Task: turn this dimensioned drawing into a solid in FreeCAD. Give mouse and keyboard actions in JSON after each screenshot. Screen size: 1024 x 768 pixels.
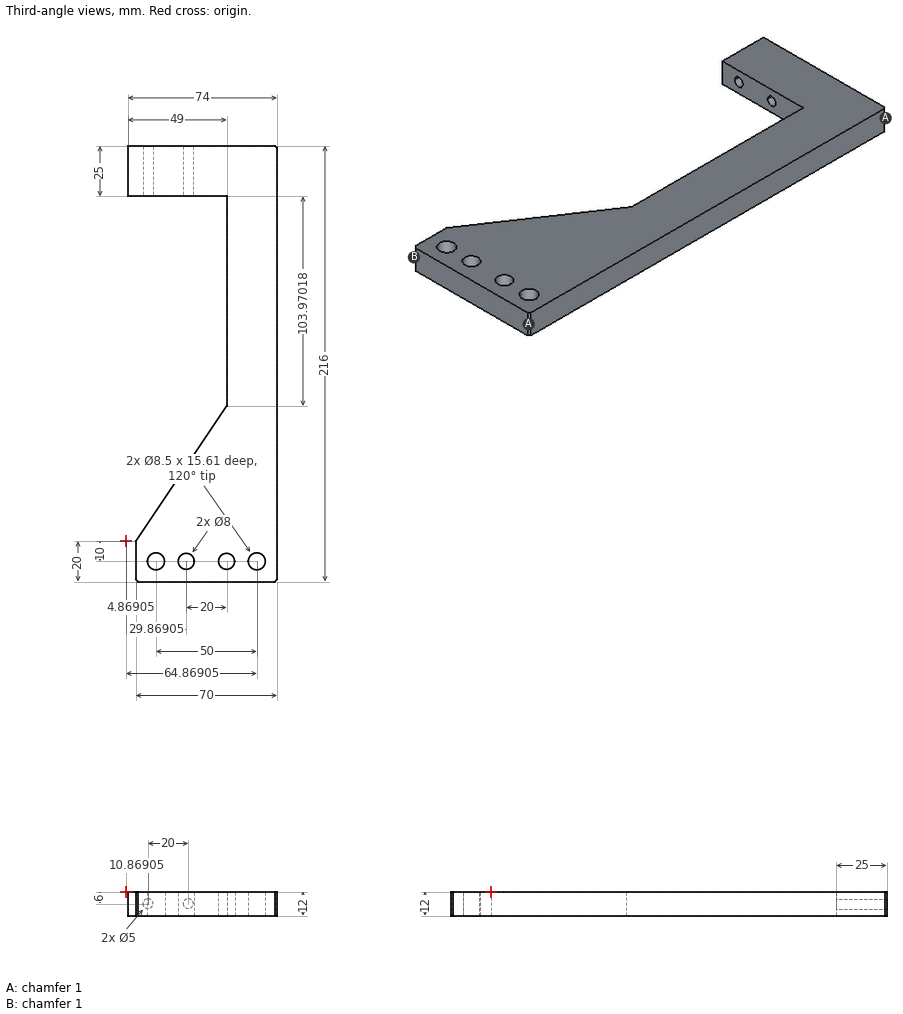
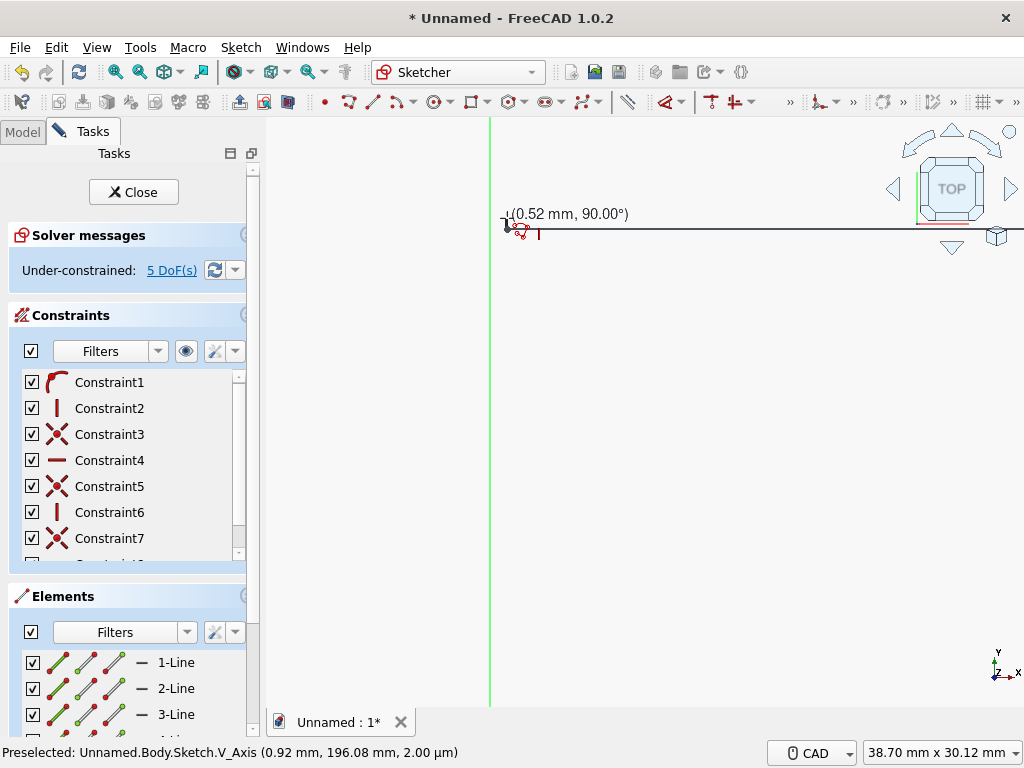
{"action": "scroll", "coordinate": [512, 220], "scroll_direction": "down", "scroll_amount": 12}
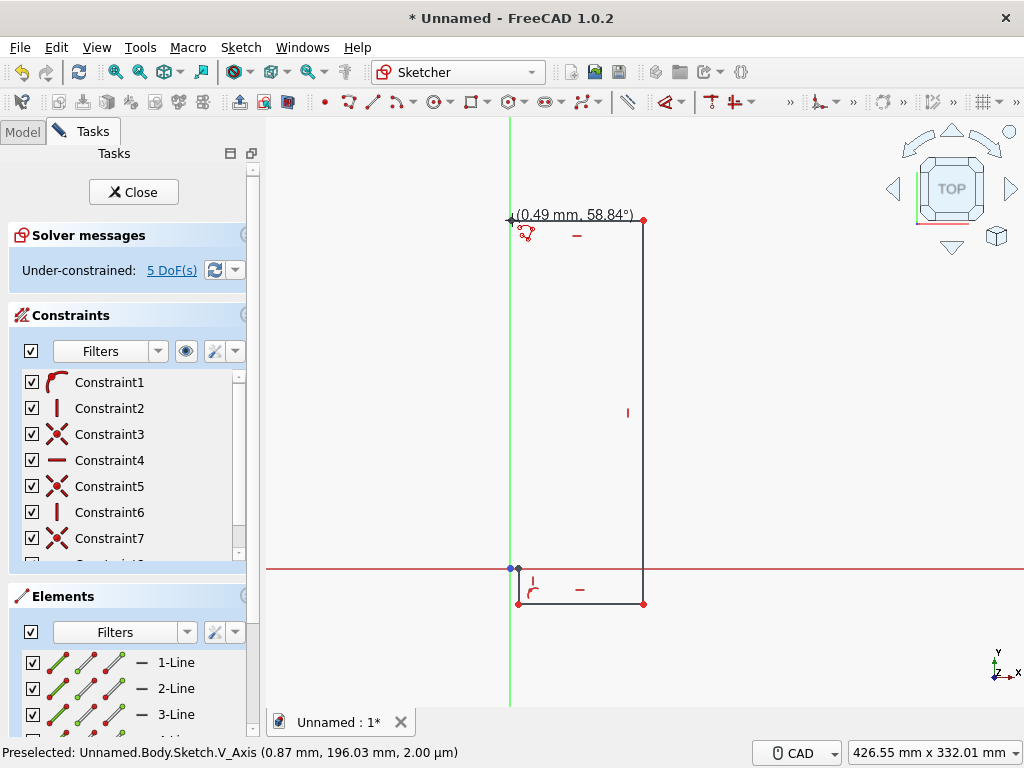
{"action": "scroll", "coordinate": [512, 265], "scroll_direction": "up", "scroll_amount": 12}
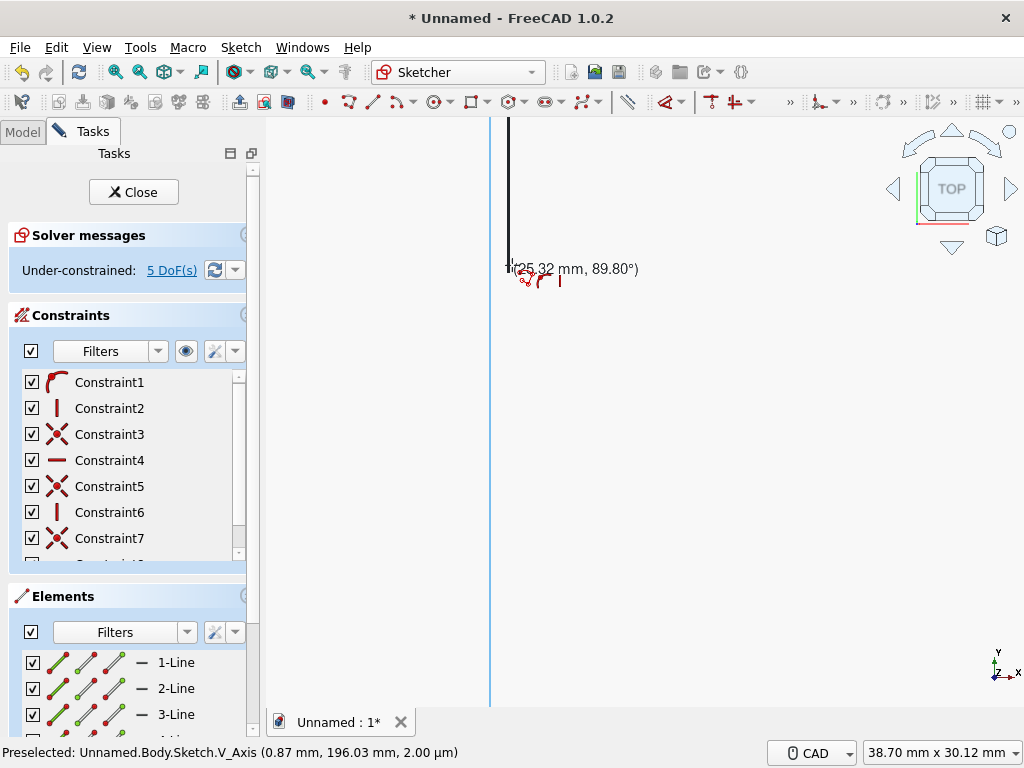
{"action": "left_click", "coordinate": [507, 259]}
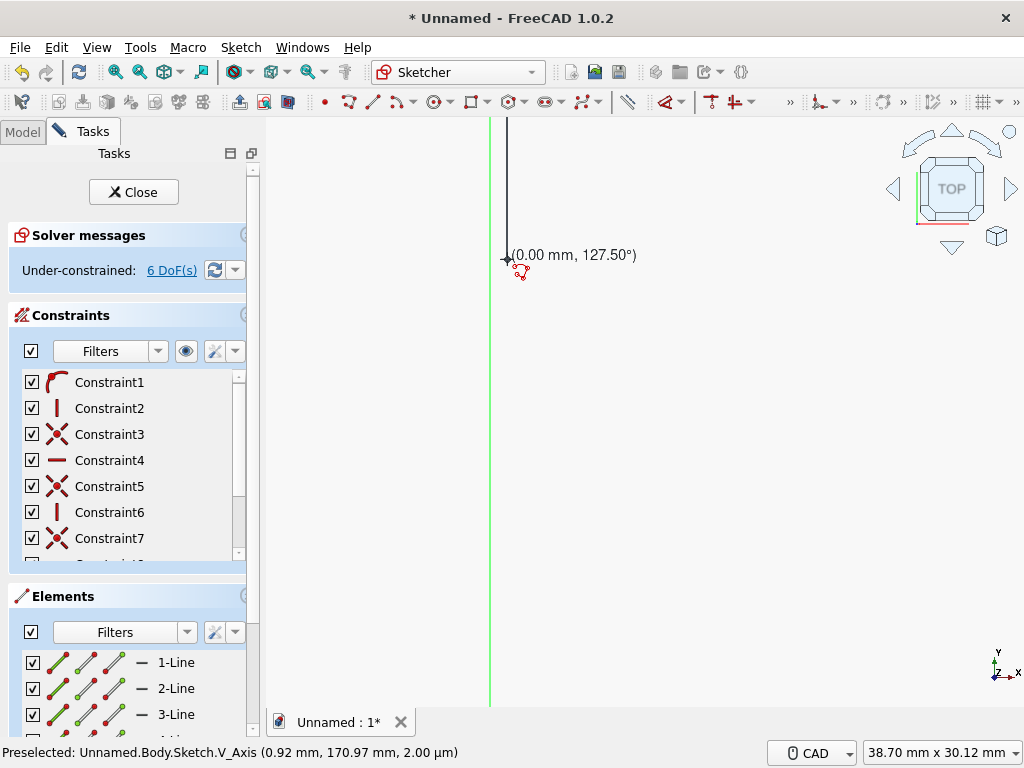
{"action": "scroll", "coordinate": [512, 265], "scroll_direction": "down", "scroll_amount": 12}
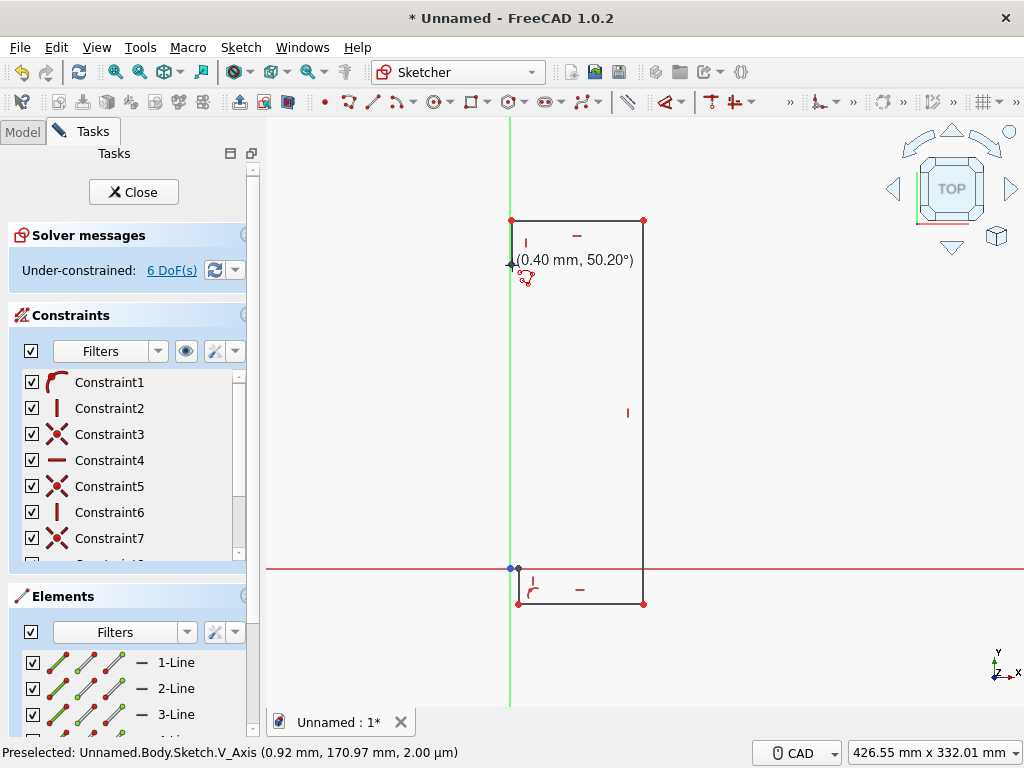
{"action": "left_click", "coordinate": [599, 265]}
{"action": "left_click", "coordinate": [599, 449]}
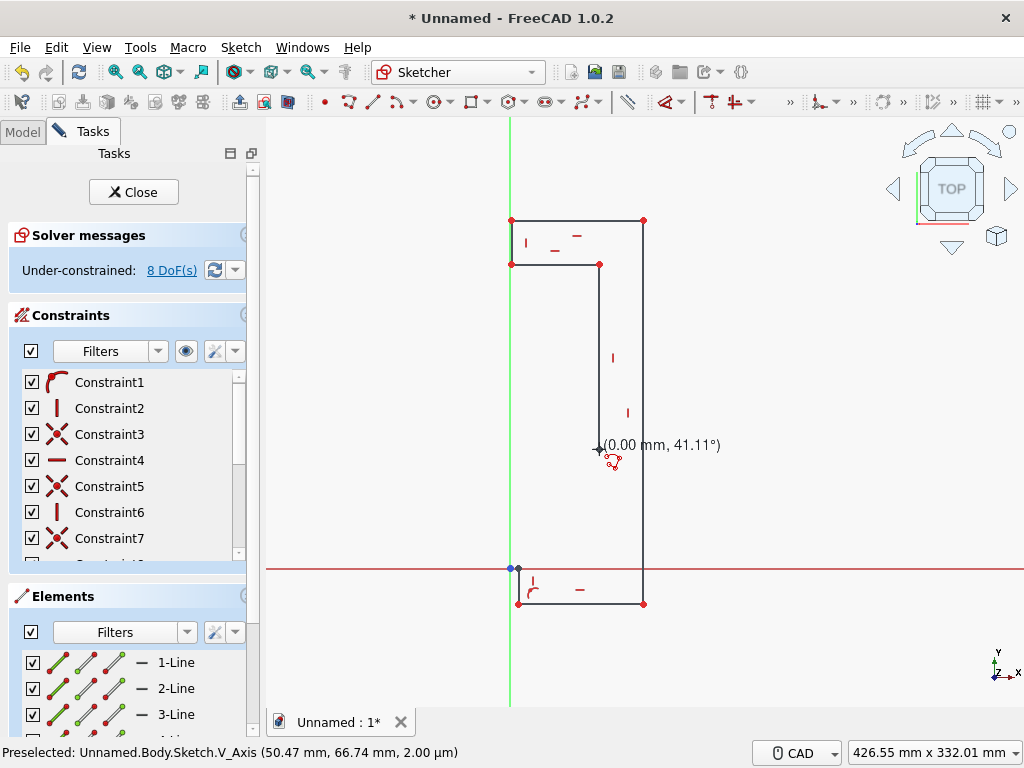
{"action": "scroll", "coordinate": [519, 569], "scroll_direction": "up", "scroll_amount": 4}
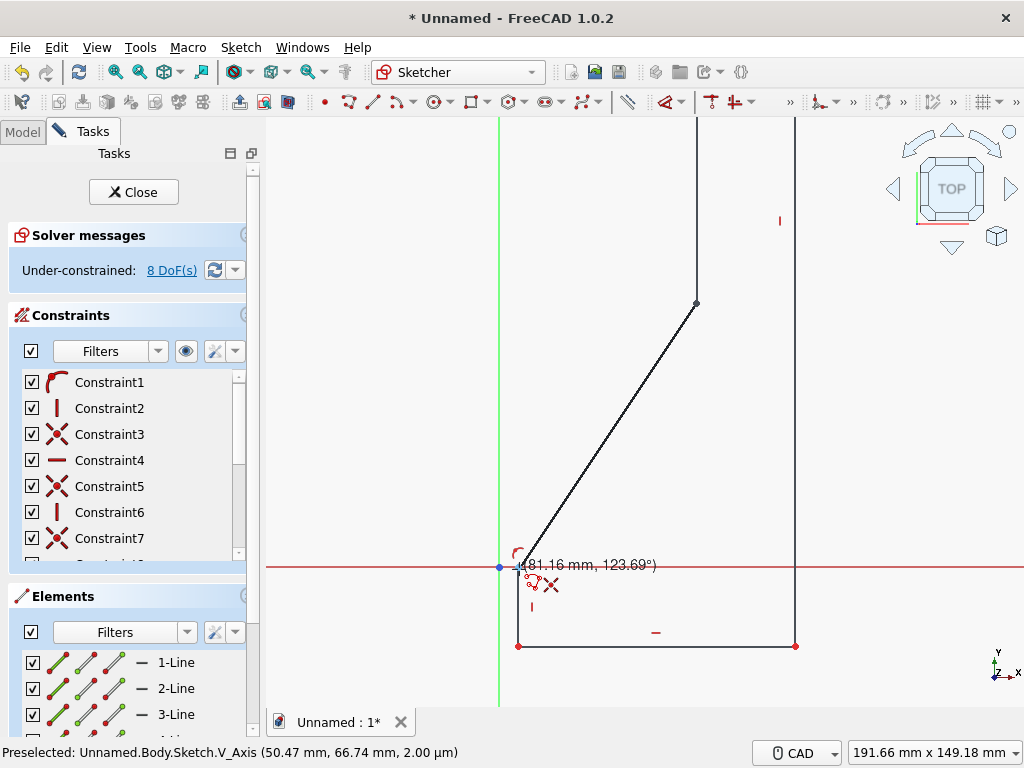
{"action": "left_click", "coordinate": [518, 567]}
{"action": "key", "text": "Escape"}
{"action": "key", "text": "Escape"}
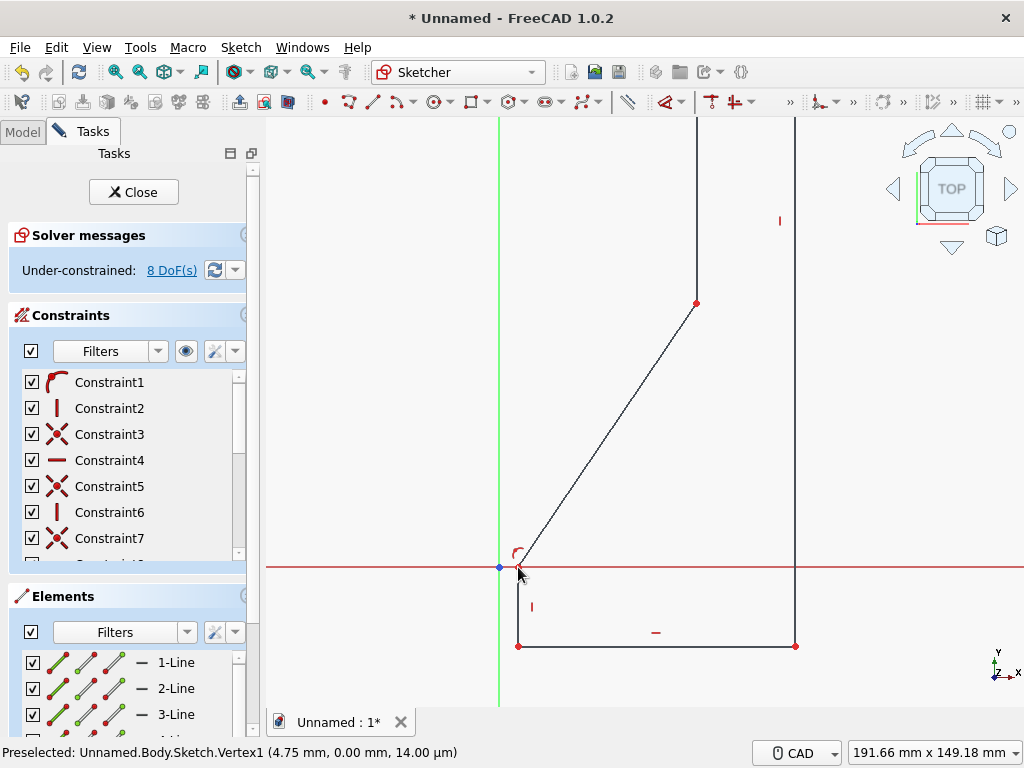
{"action": "key", "text": "d"}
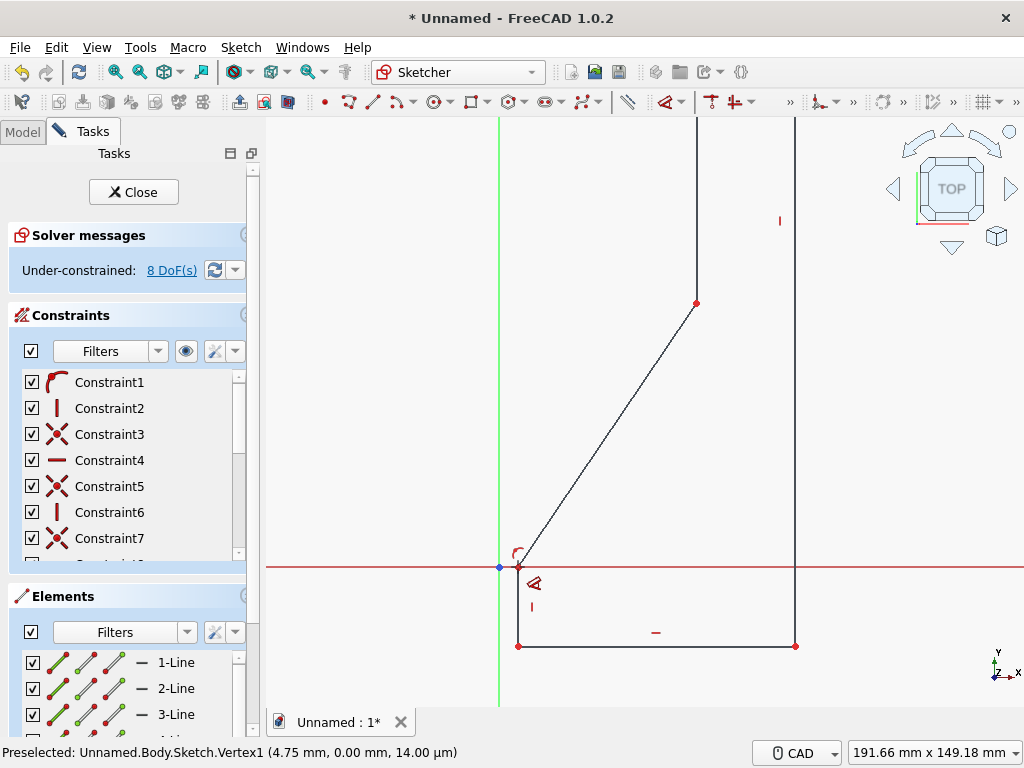
{"action": "left_click", "coordinate": [518, 591]}
{"action": "left_click", "coordinate": [484, 607]}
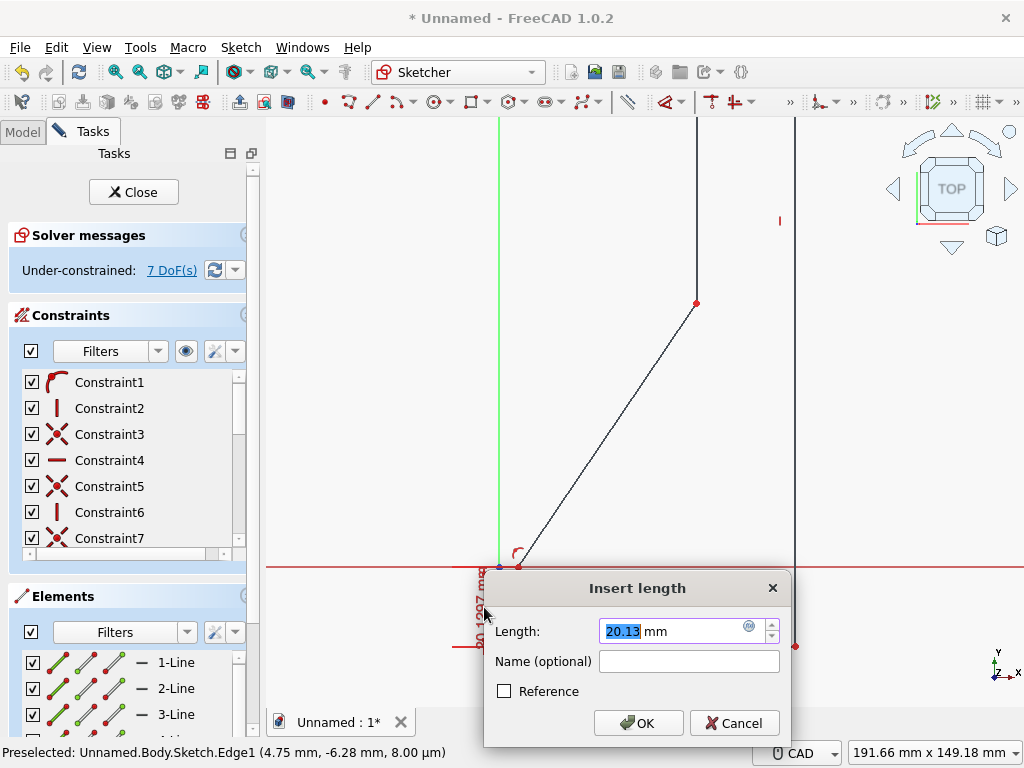
{"action": "type", "text": "20"}
{"action": "key", "text": "Return"}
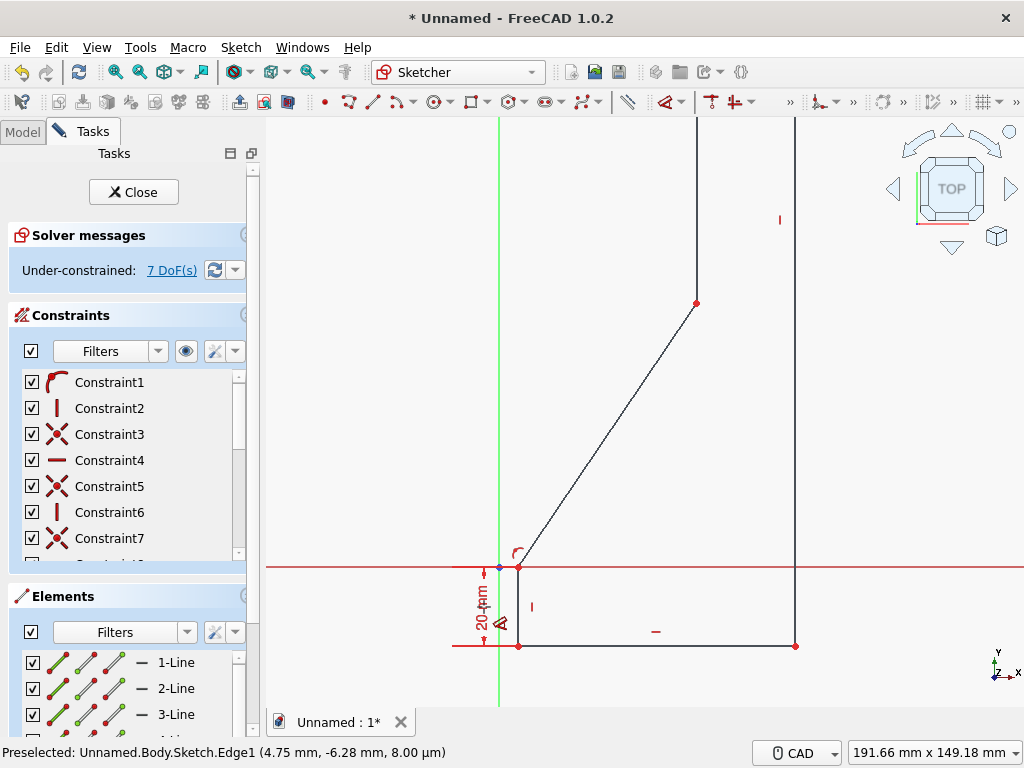
{"action": "left_click", "coordinate": [601, 646]}
{"action": "left_click", "coordinate": [656, 612]}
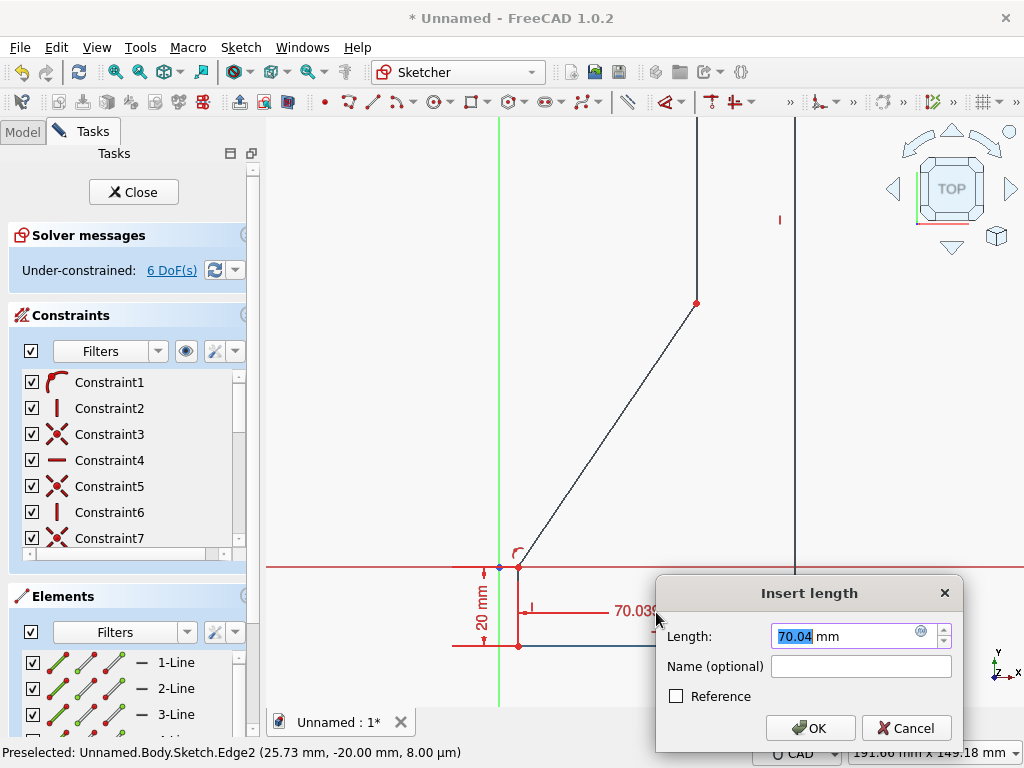
{"action": "type", "text": "70"}
{"action": "key", "text": "Return"}